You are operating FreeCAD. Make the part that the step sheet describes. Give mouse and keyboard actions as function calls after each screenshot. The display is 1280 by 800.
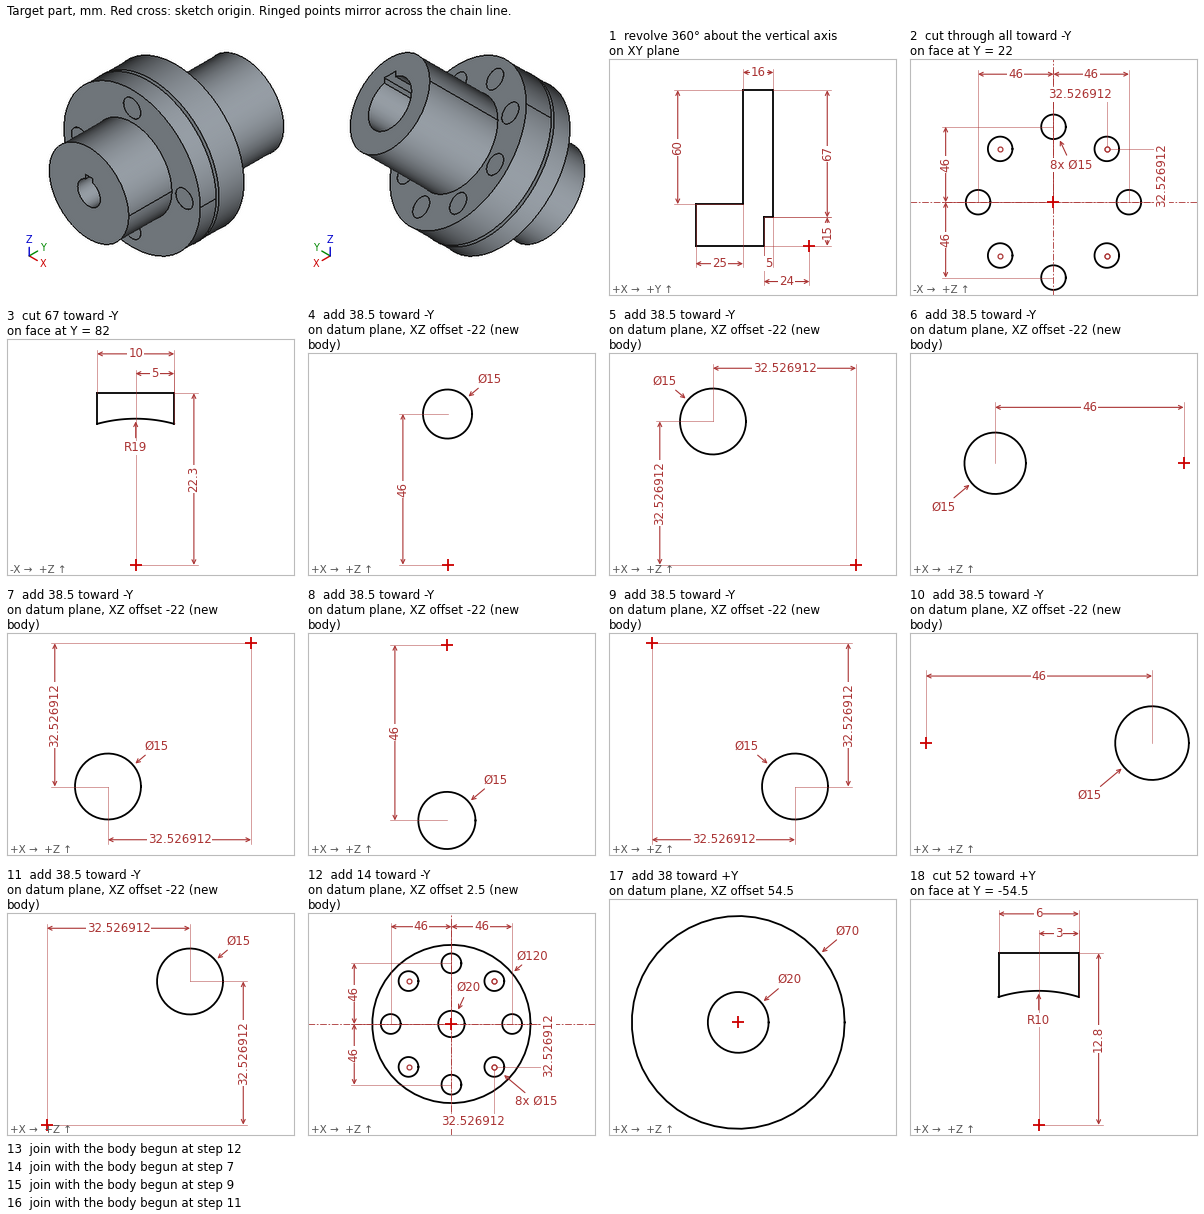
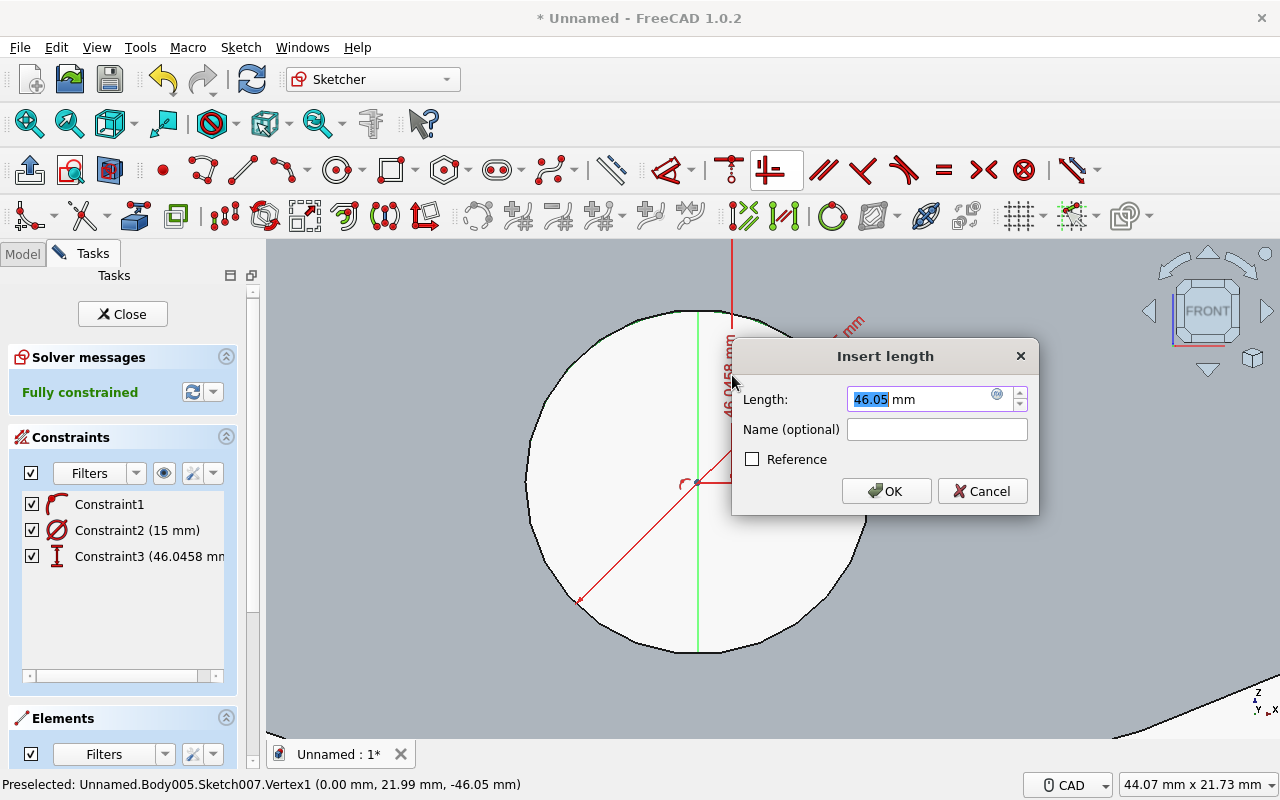
text(46)
key(Return)
key(Escape)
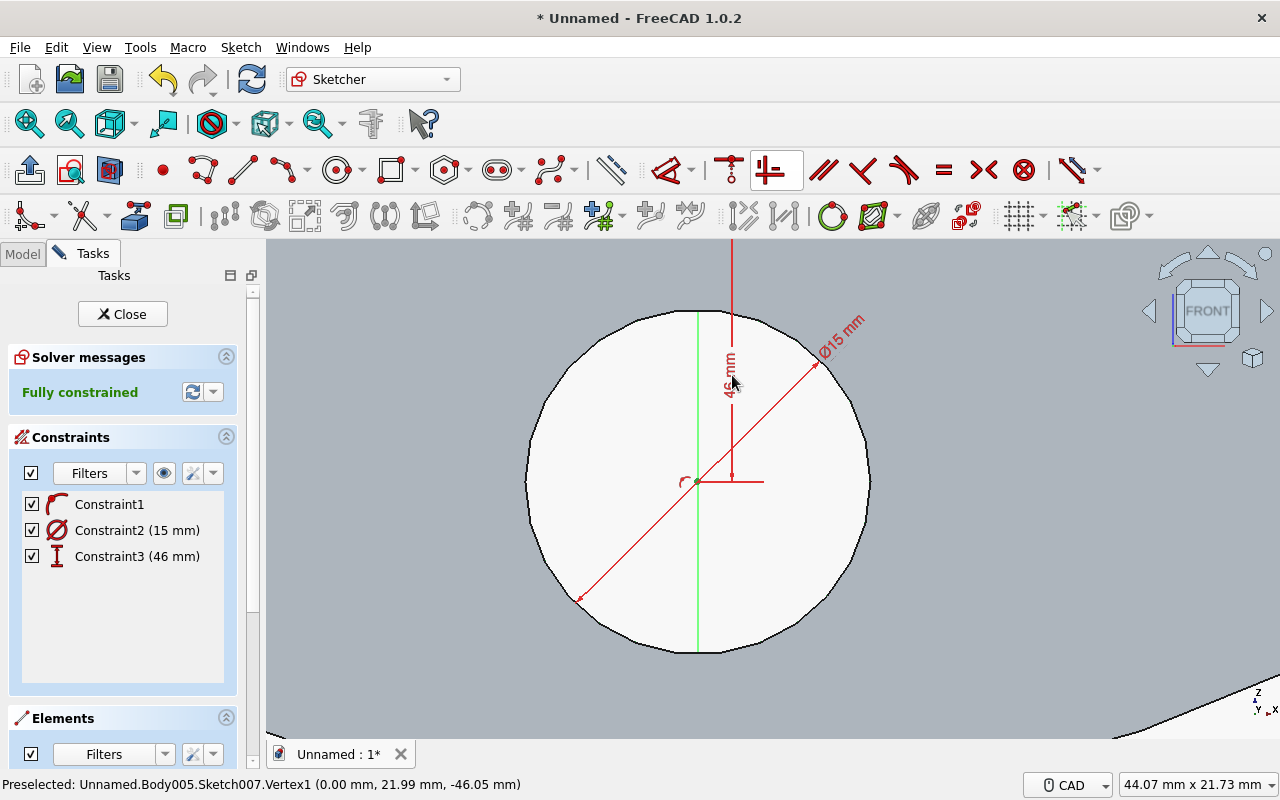
click(123, 314)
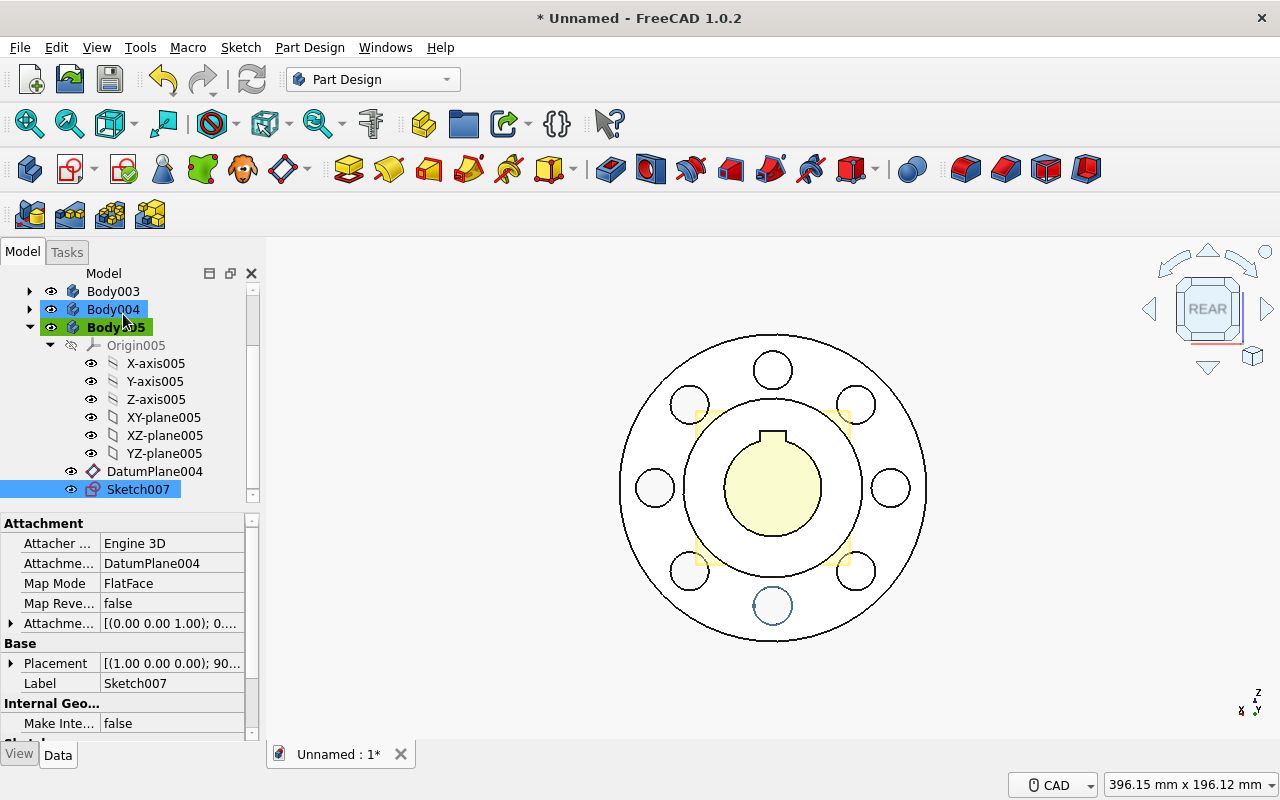
click(350, 170)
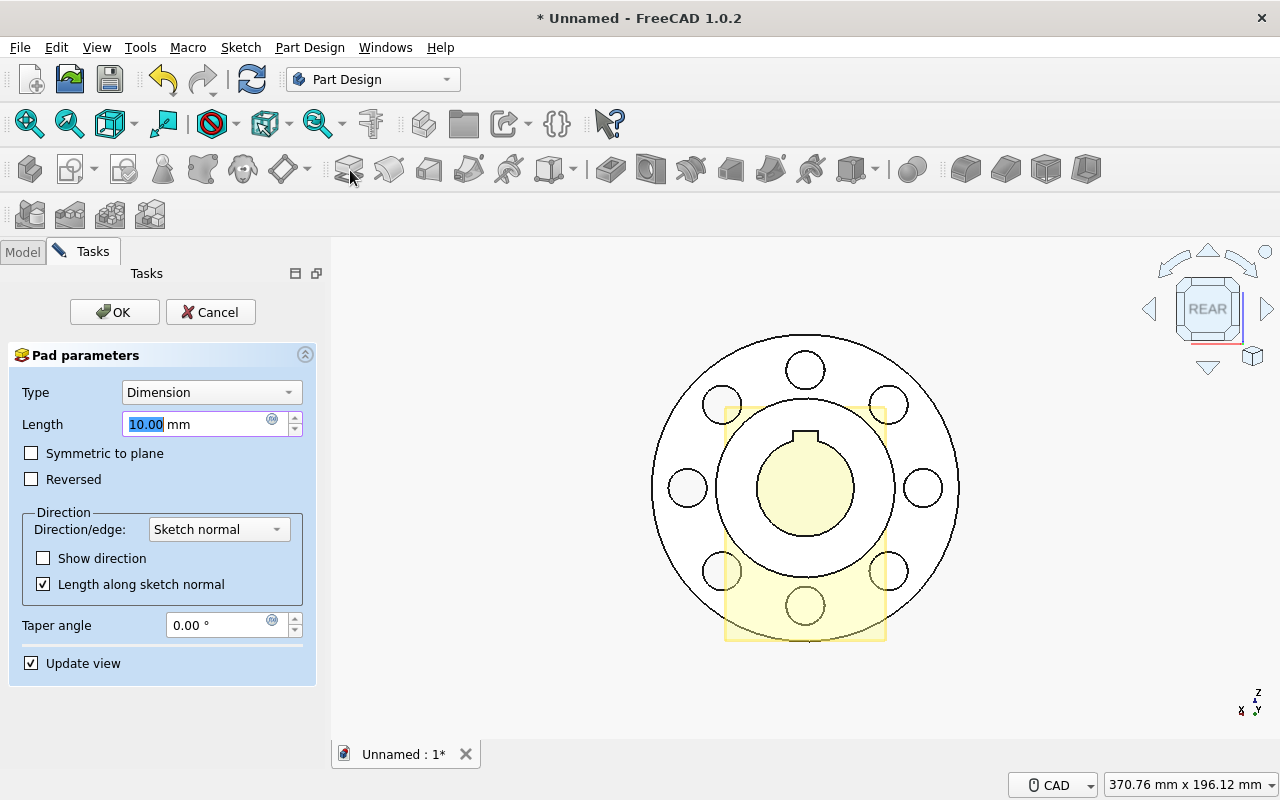
text(38.5)
key(Tab)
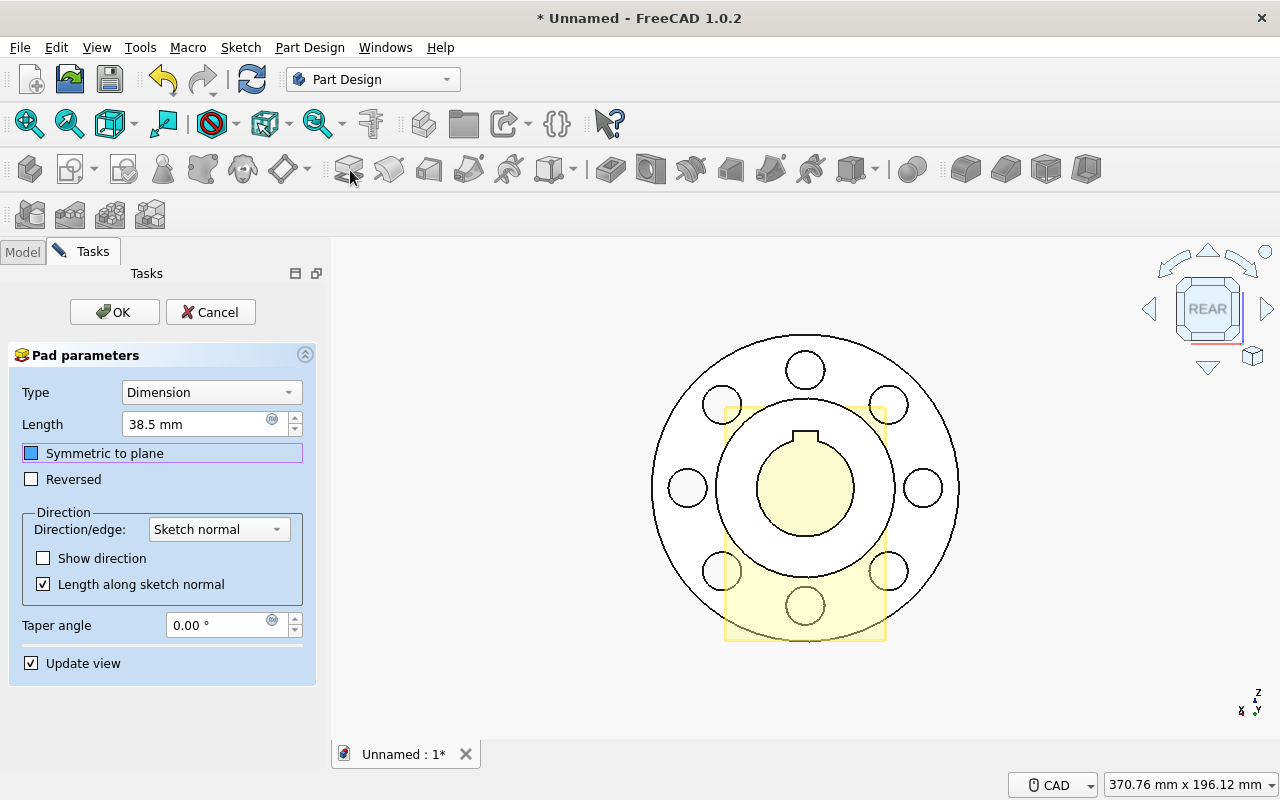
click(115, 312)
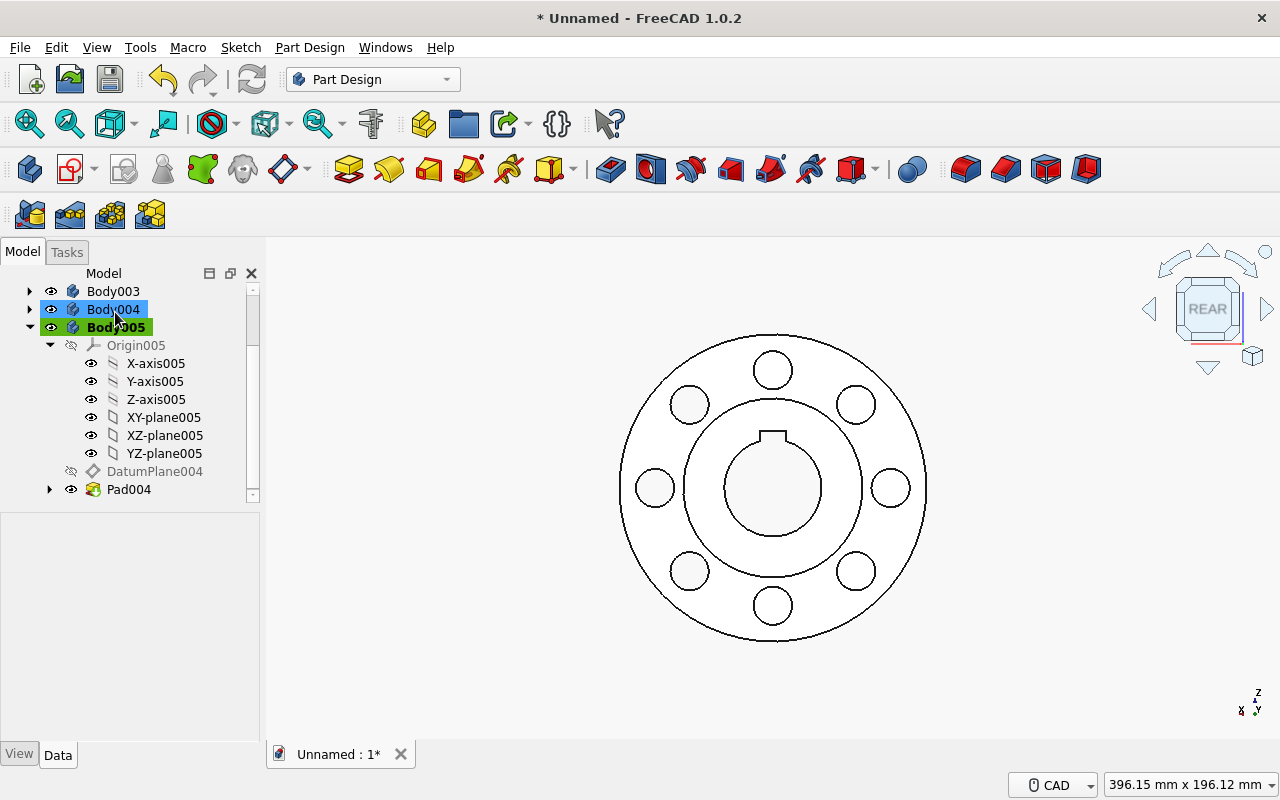
click(30, 124)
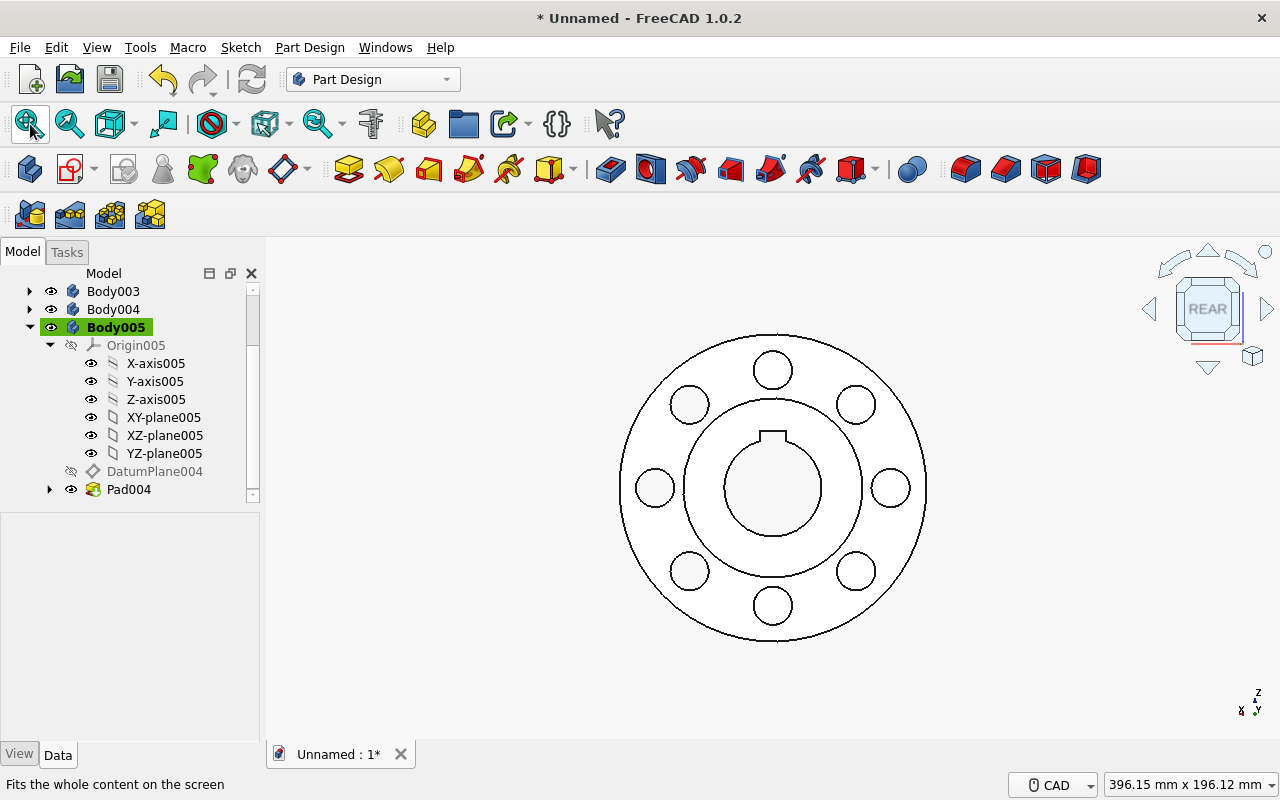
click(30, 170)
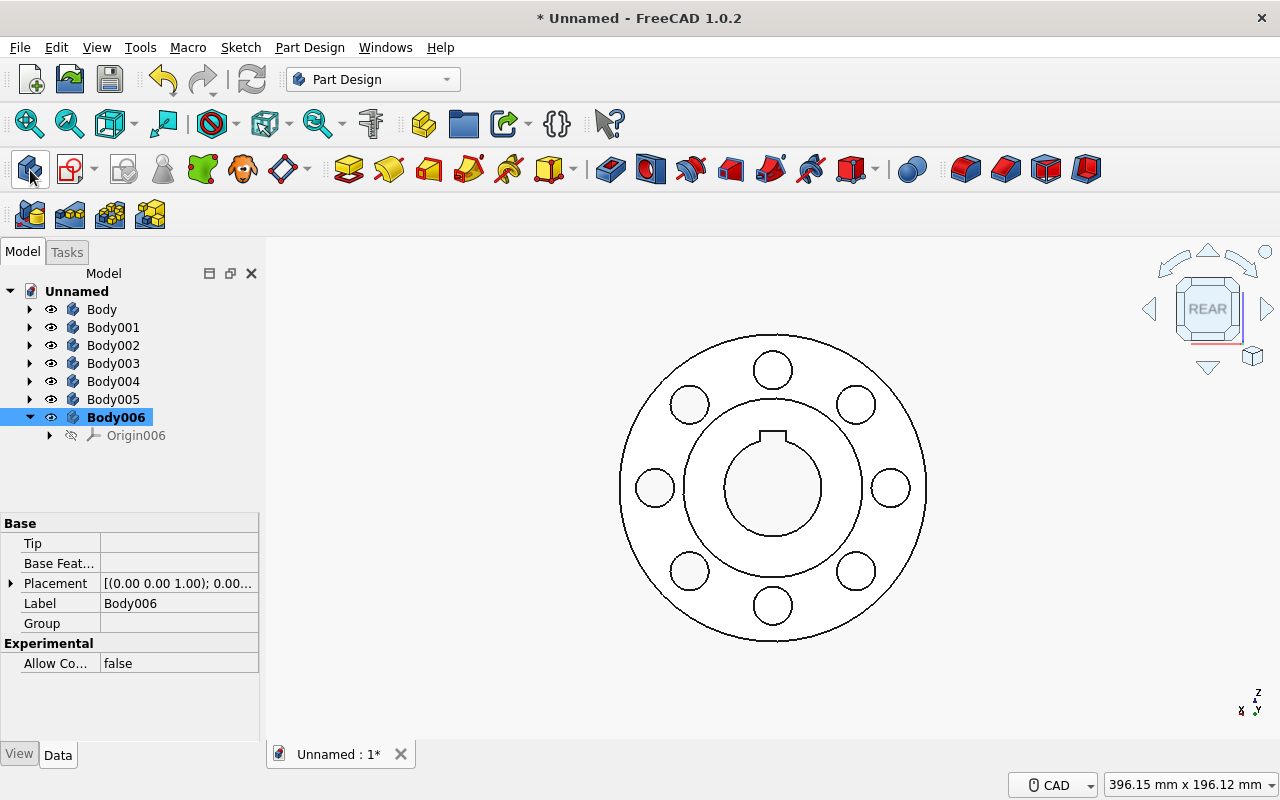
click(50, 435)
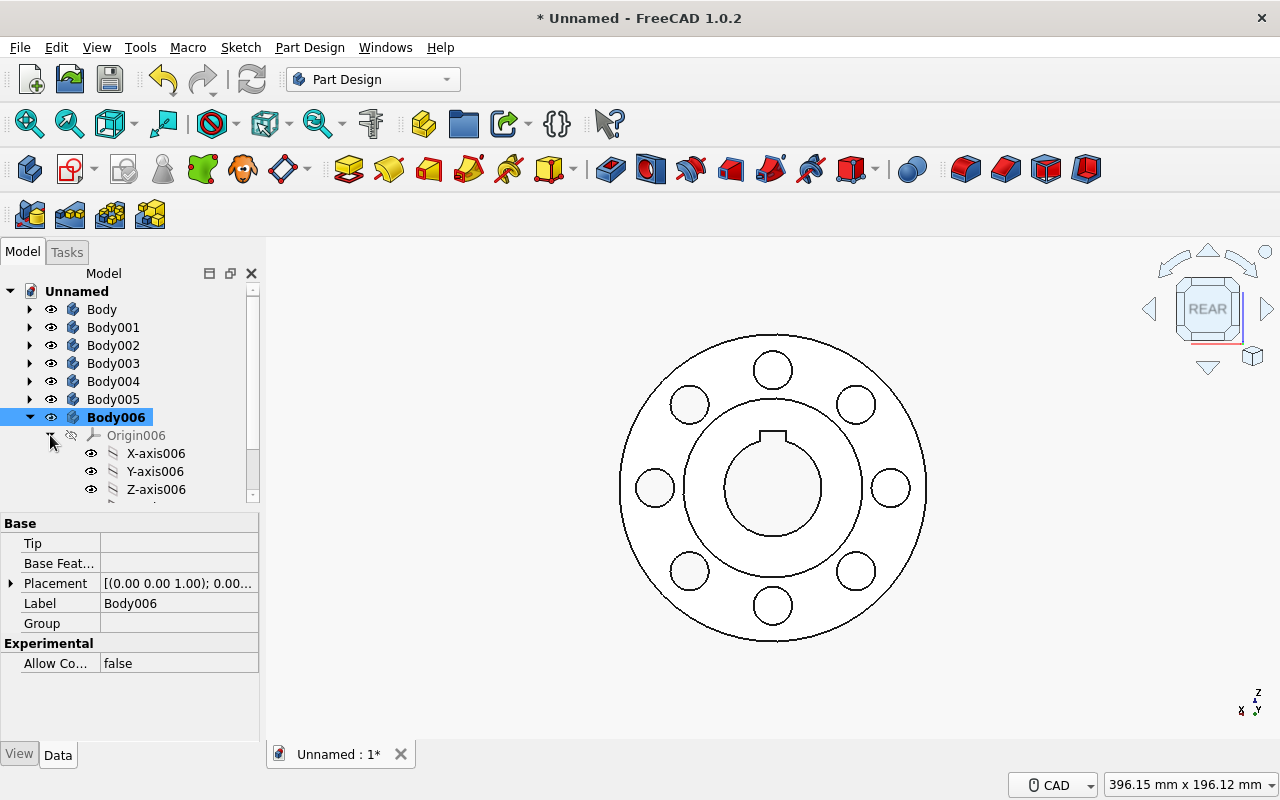
scroll(100, 395, down, 3)